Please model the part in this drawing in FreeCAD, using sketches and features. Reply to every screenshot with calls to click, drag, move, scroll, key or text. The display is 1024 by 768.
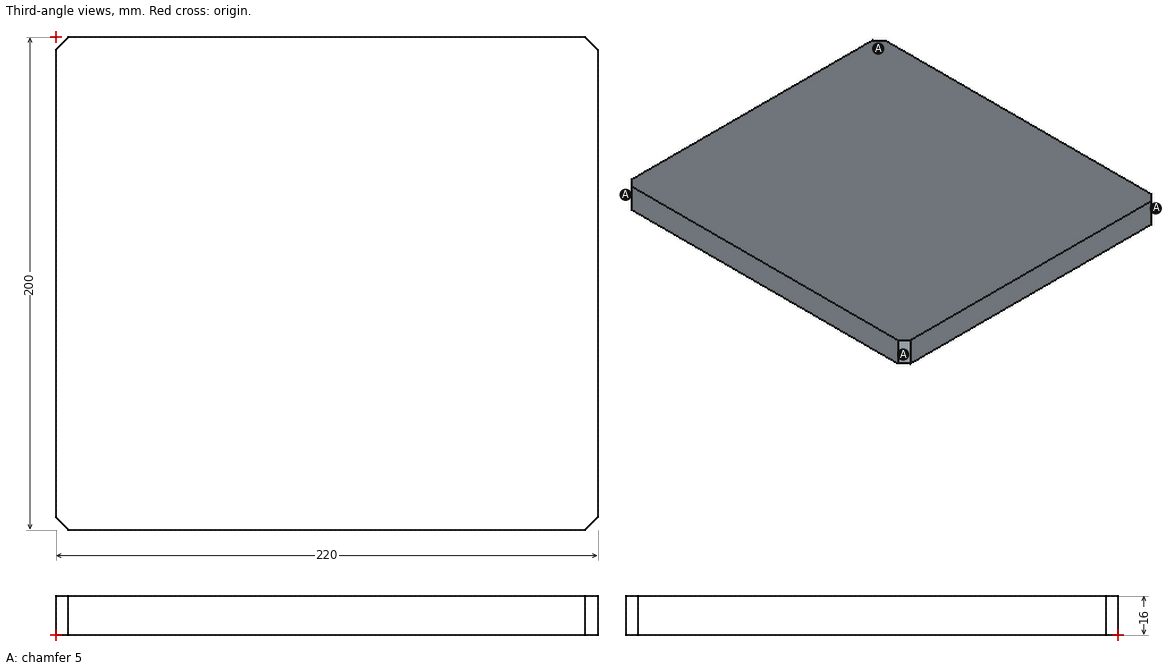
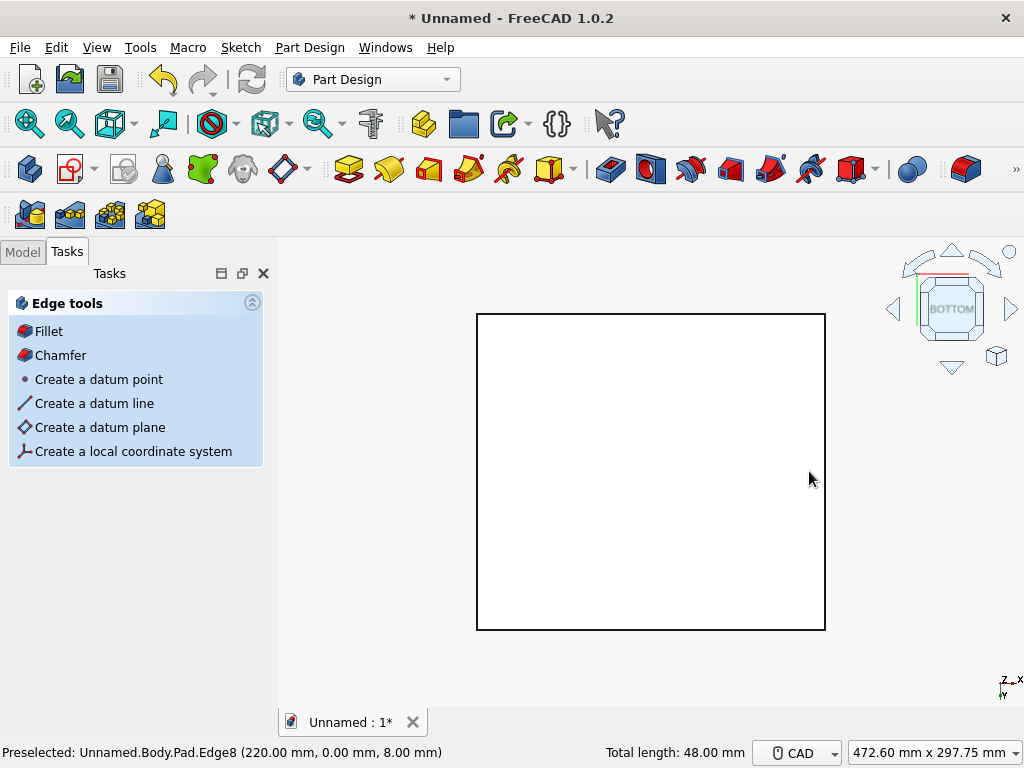
key(4)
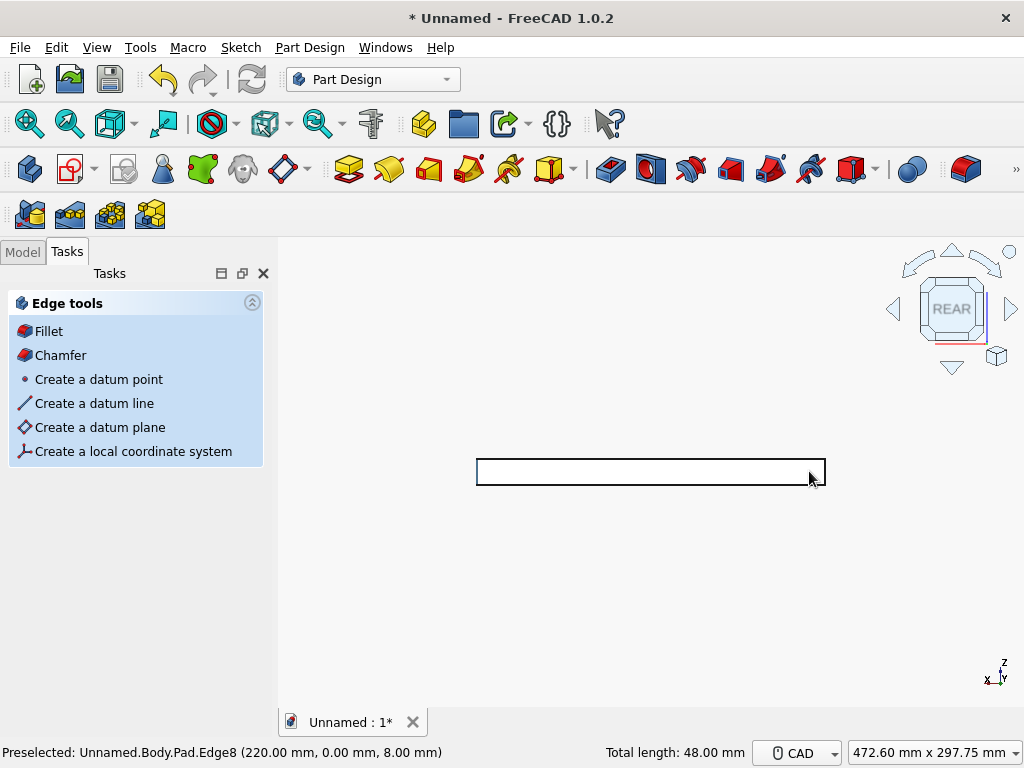
click(825, 471, ctrl)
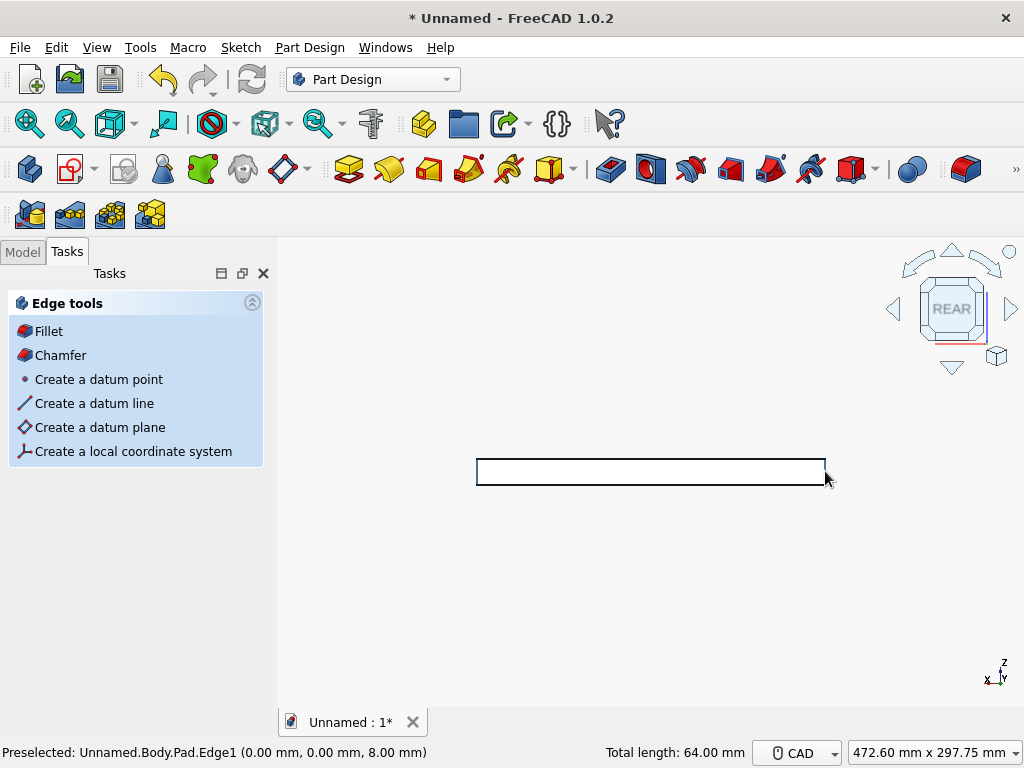
click(136, 355)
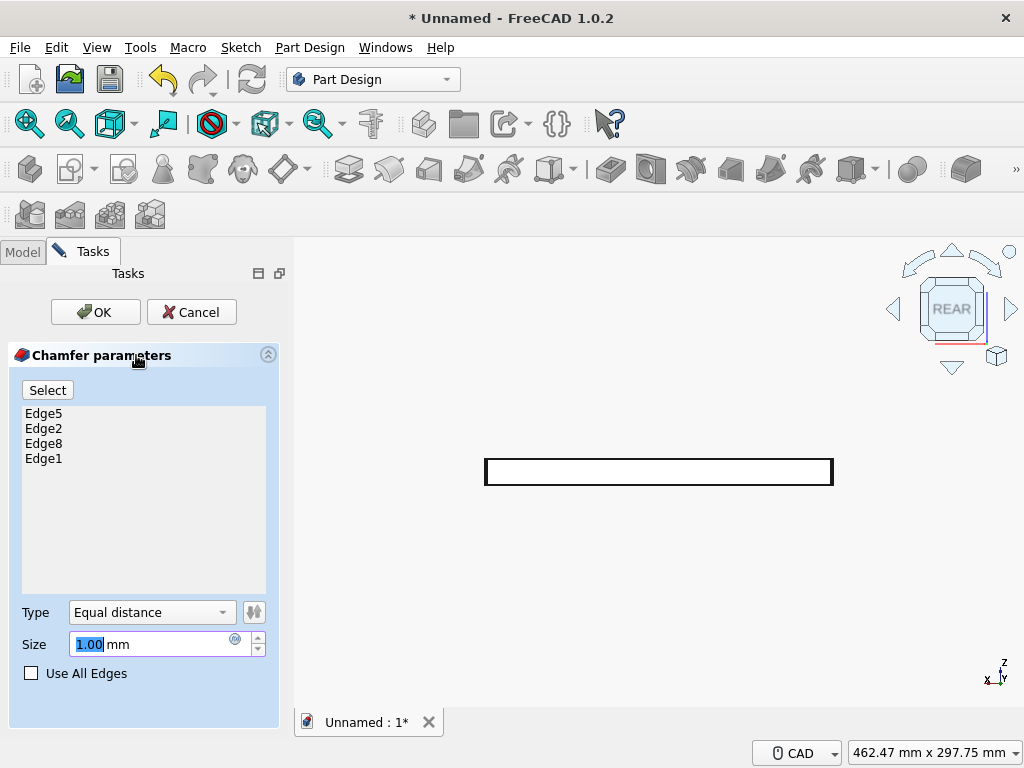
text(5)
key(Tab)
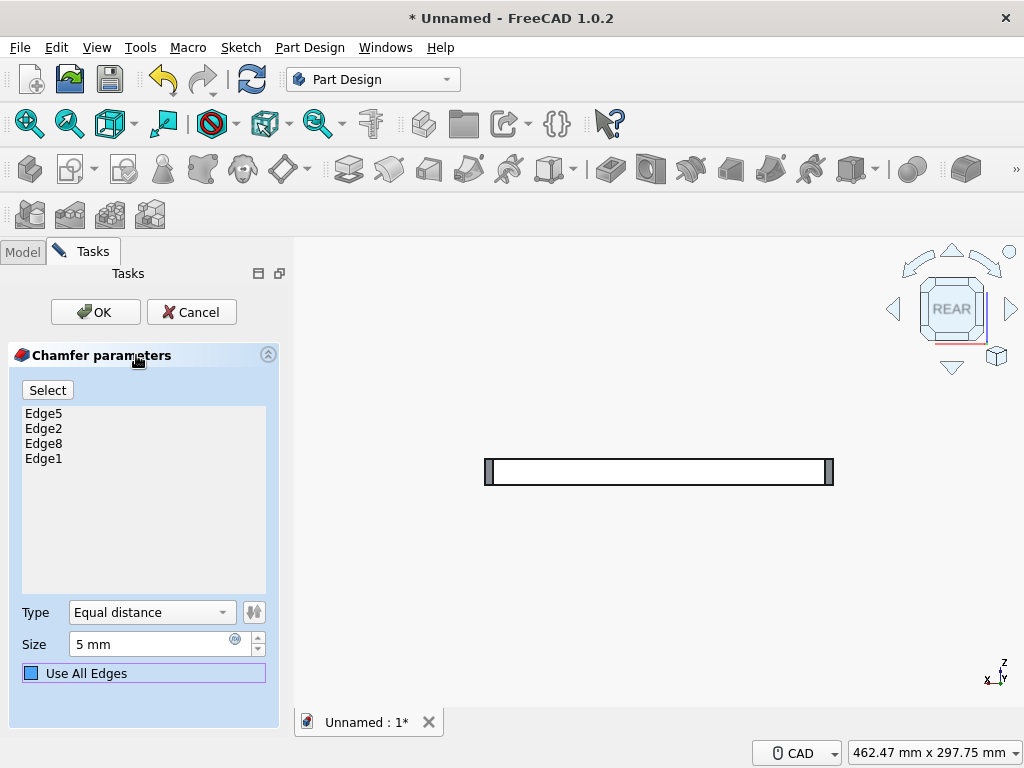
click(96, 312)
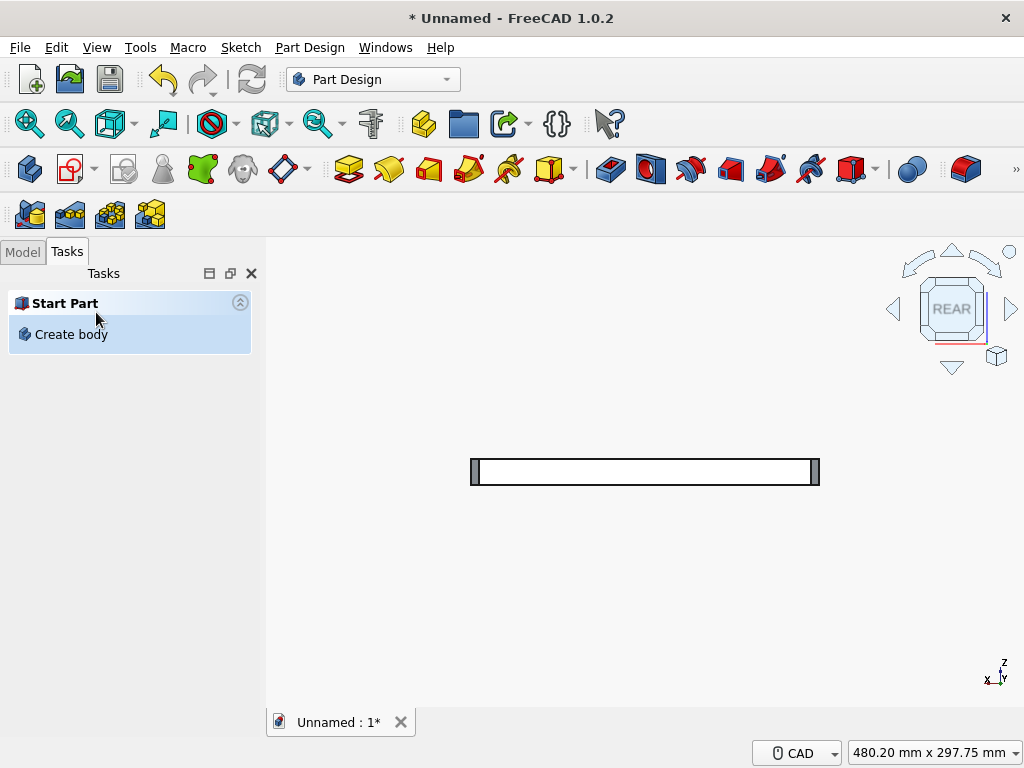
key(0)